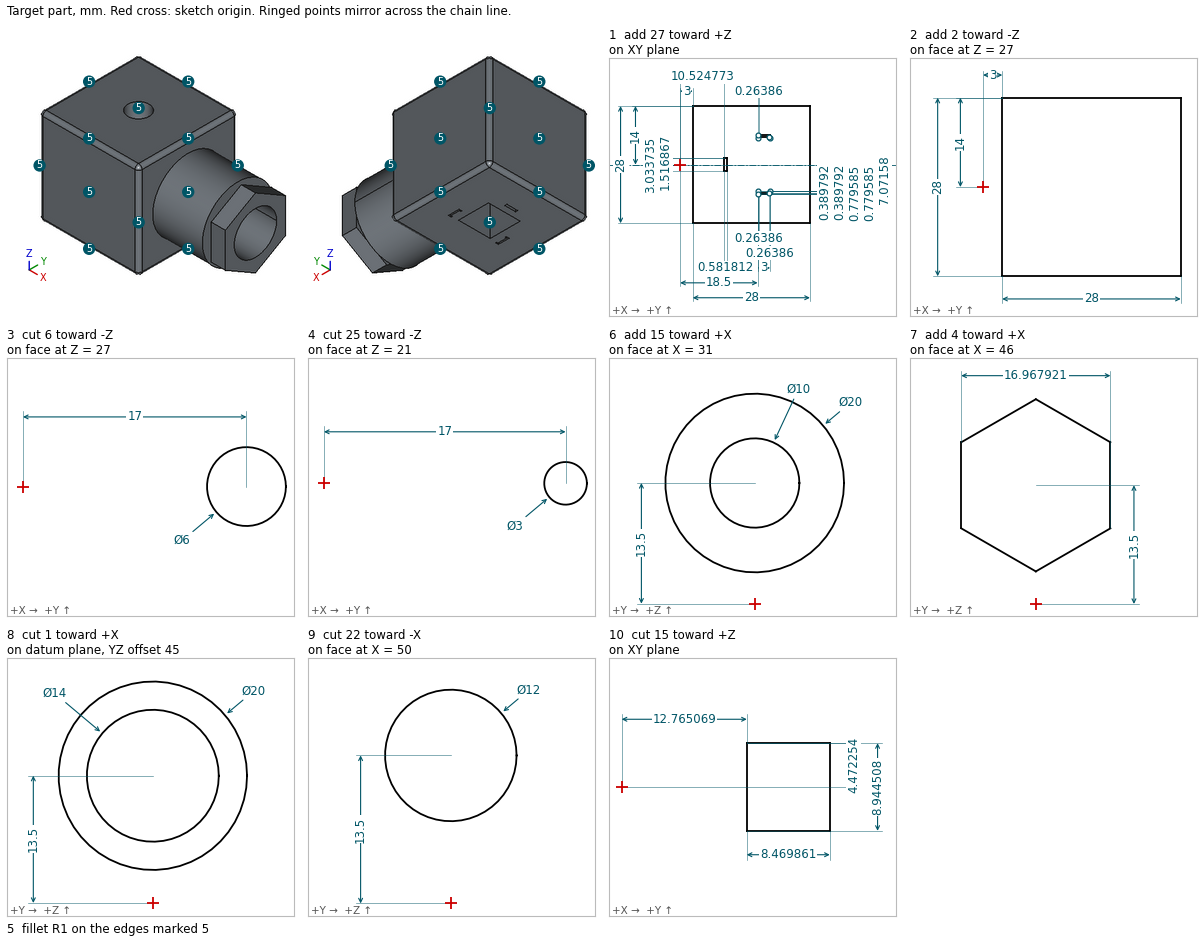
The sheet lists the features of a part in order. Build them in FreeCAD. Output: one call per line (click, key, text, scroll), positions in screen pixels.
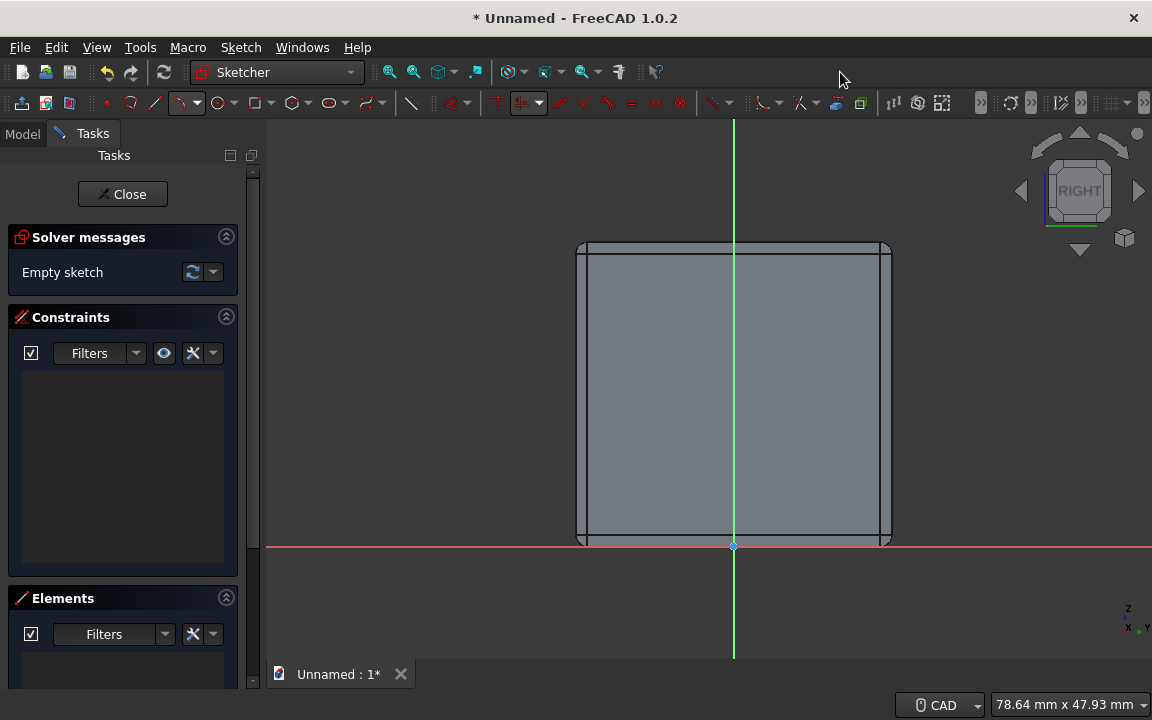
click(218, 104)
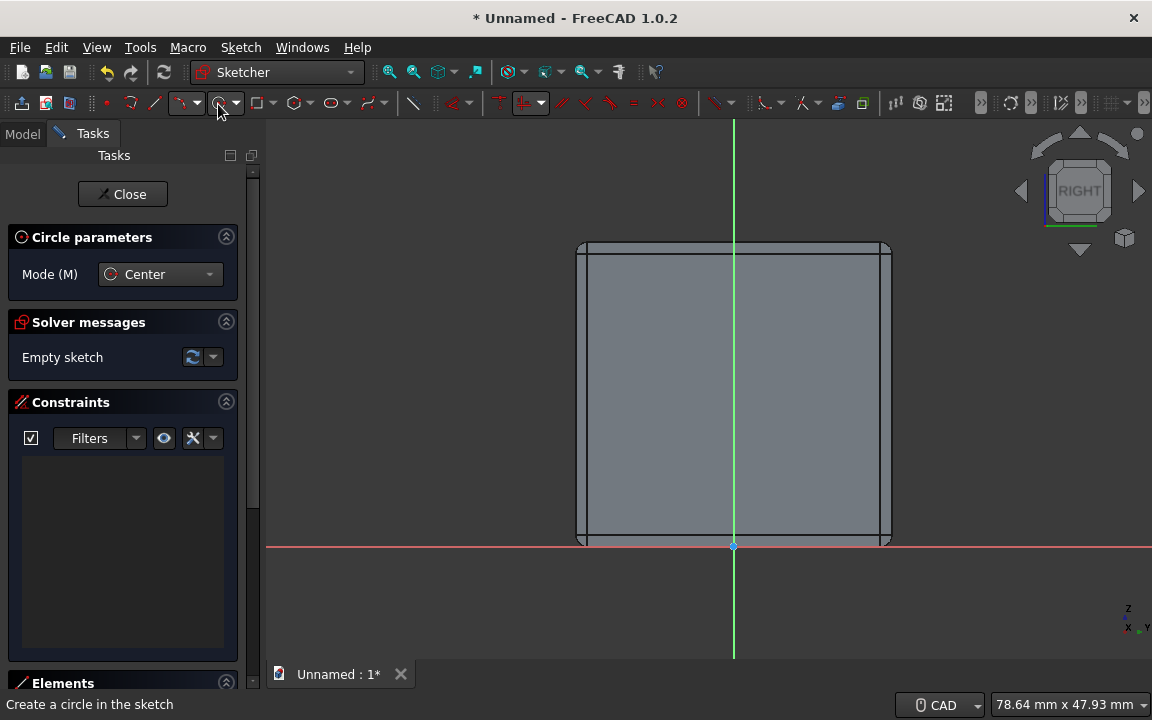
click(734, 394)
click(814, 315)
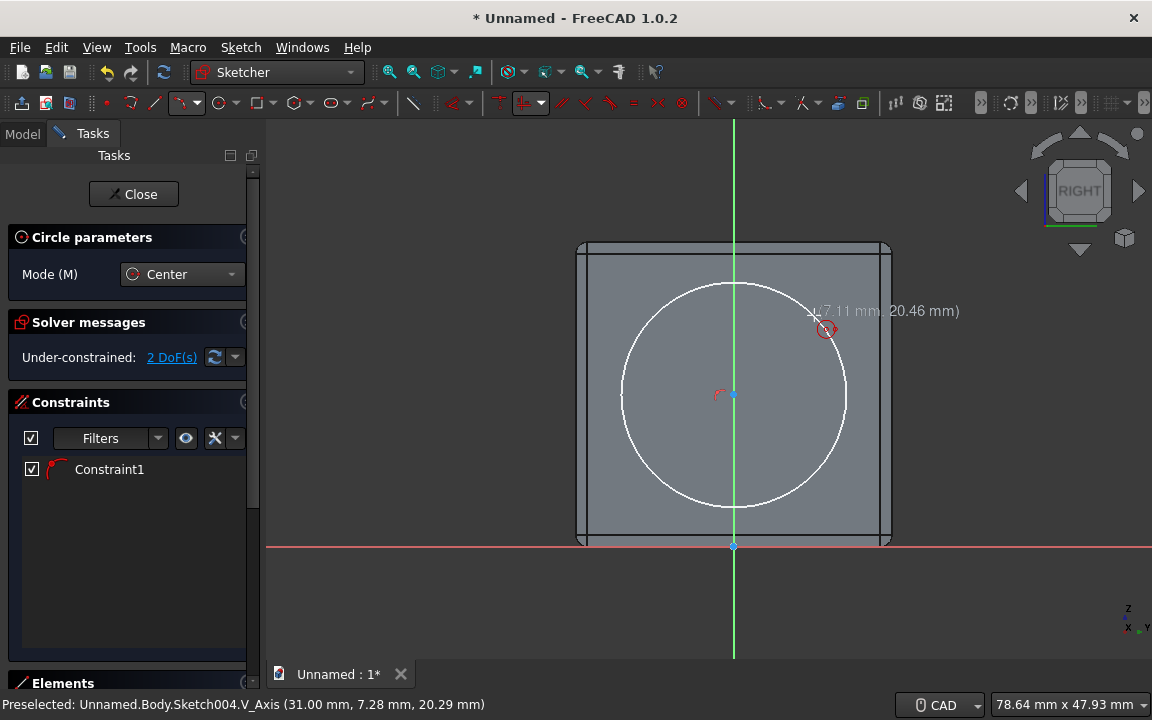
click(734, 395)
click(774, 355)
key(Escape)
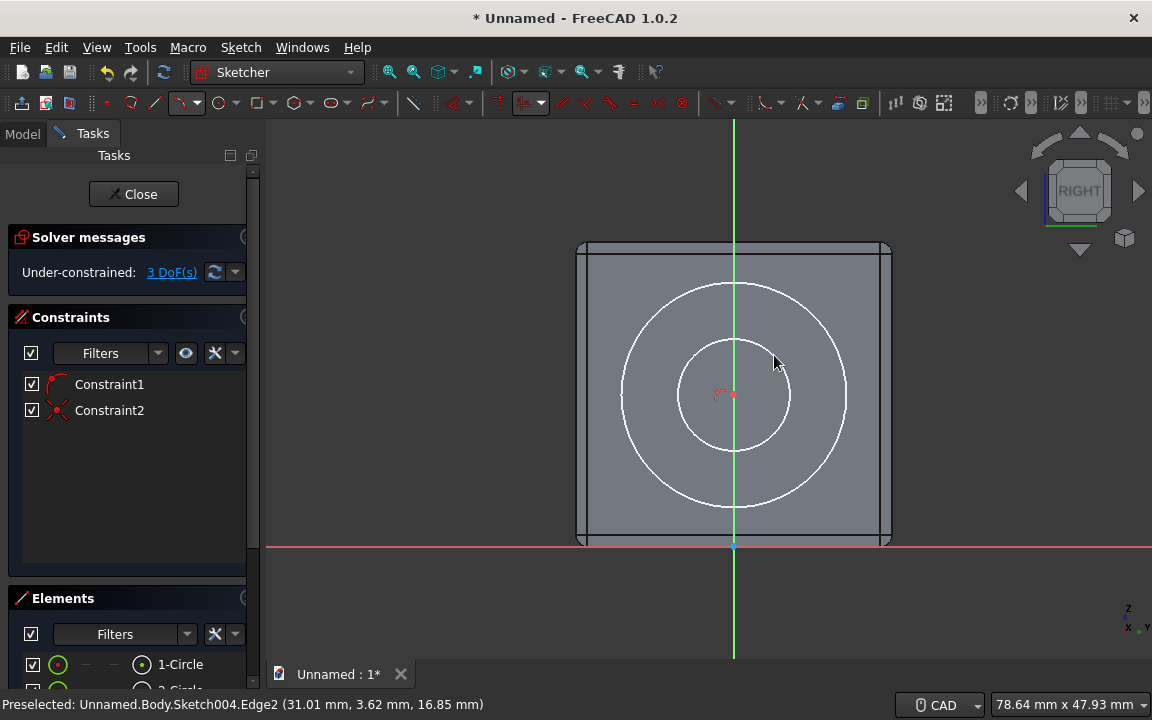
click(452, 104)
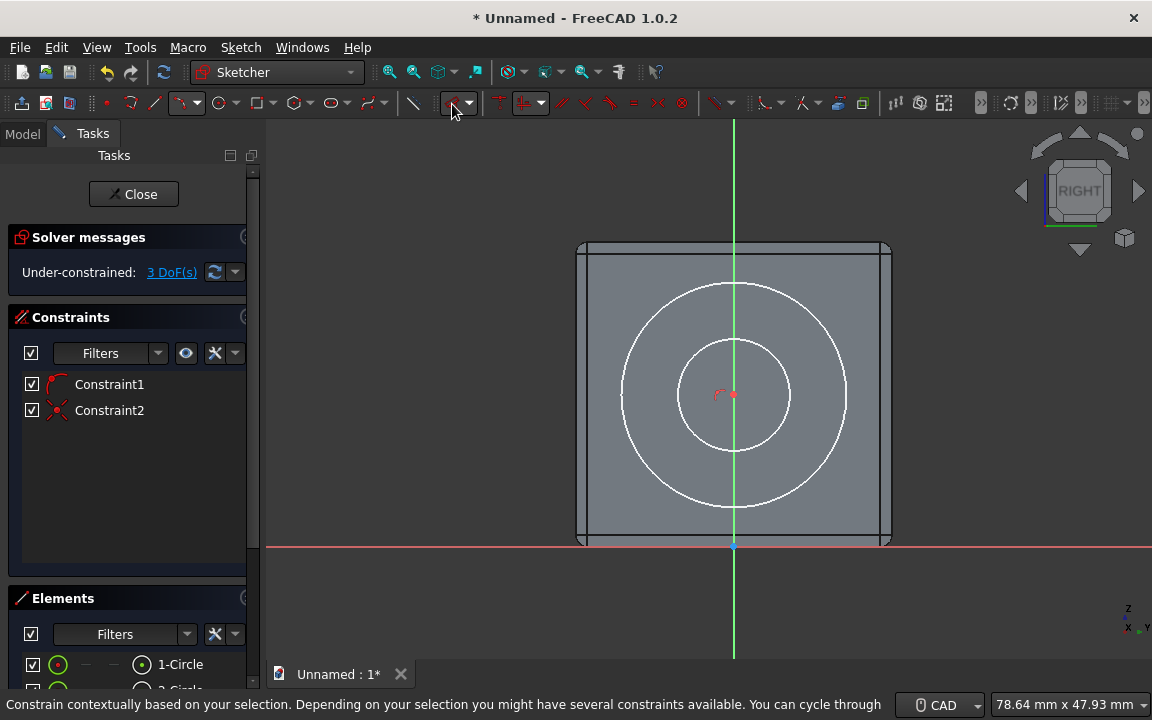
click(813, 315)
click(835, 292)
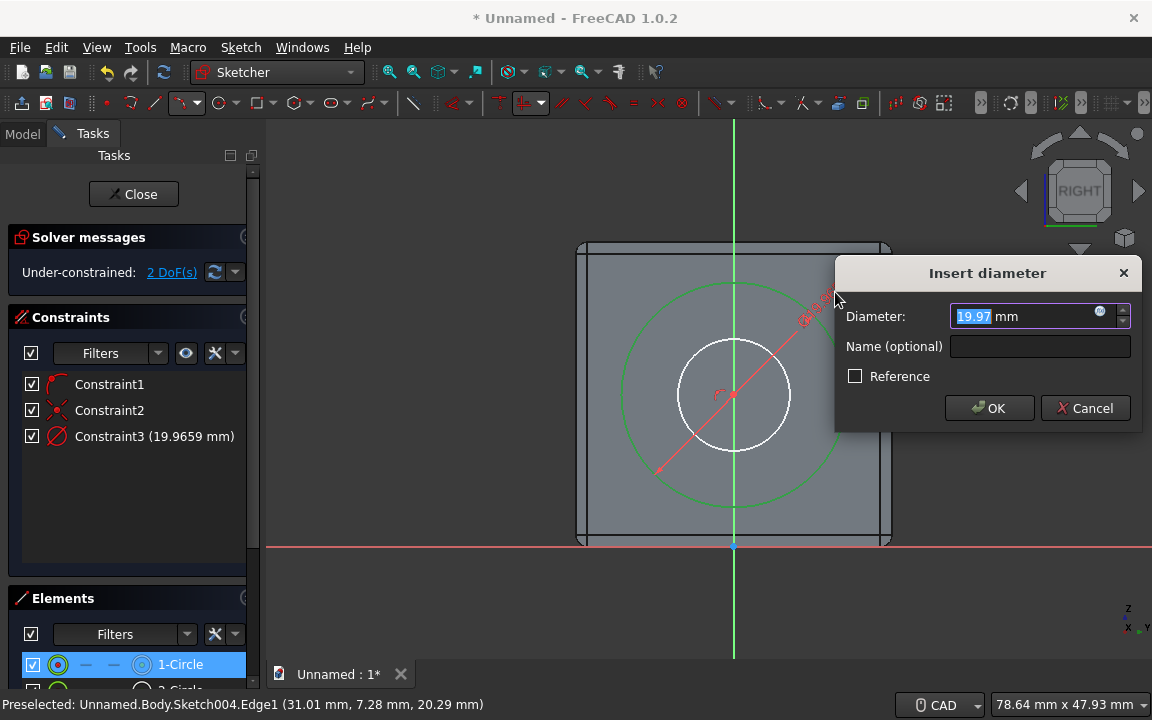
text(20)
key(Return)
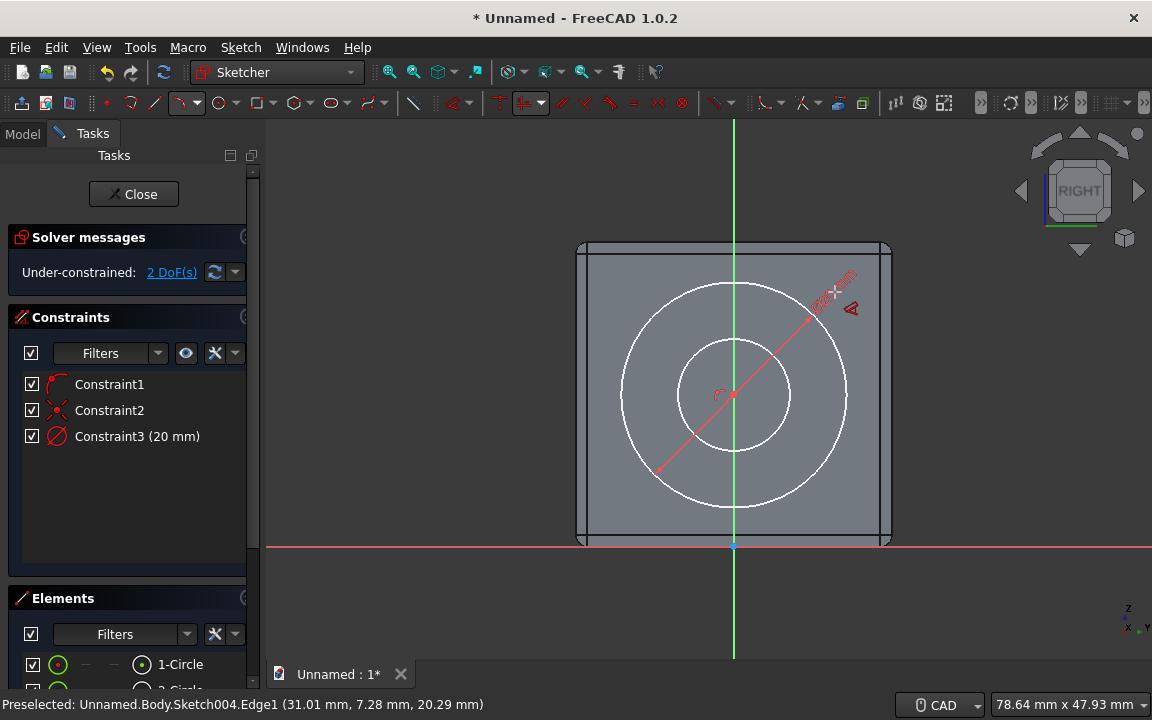
click(773, 355)
click(795, 332)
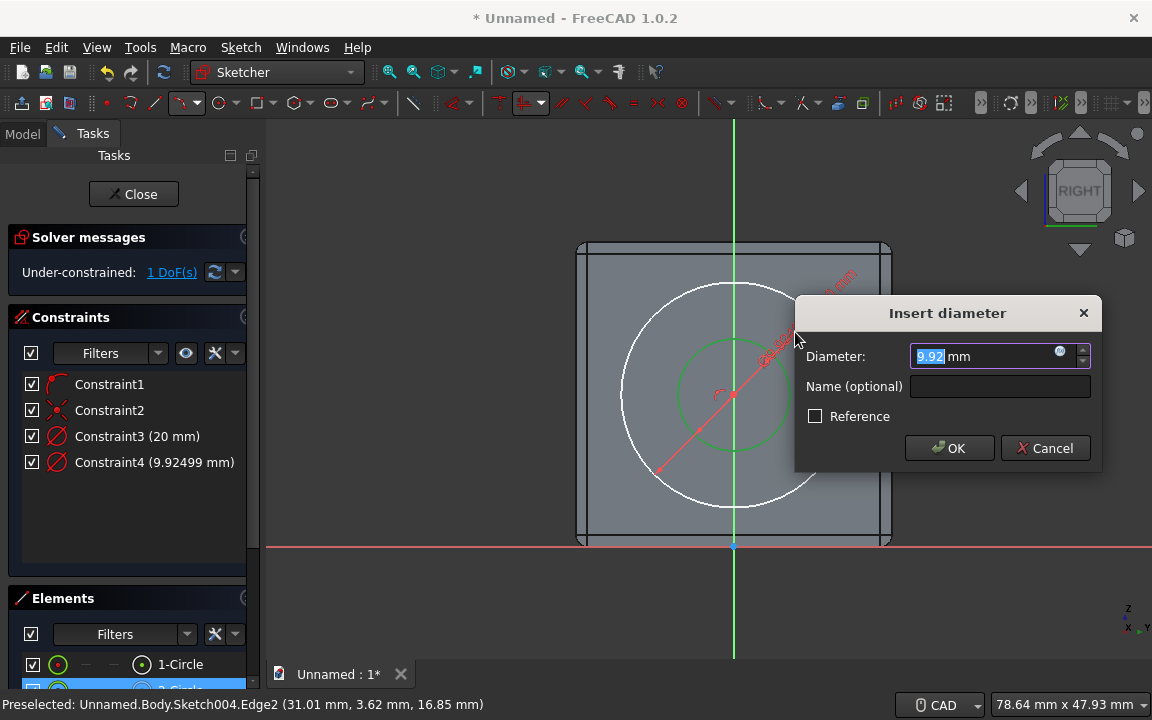
text(10)
key(Return)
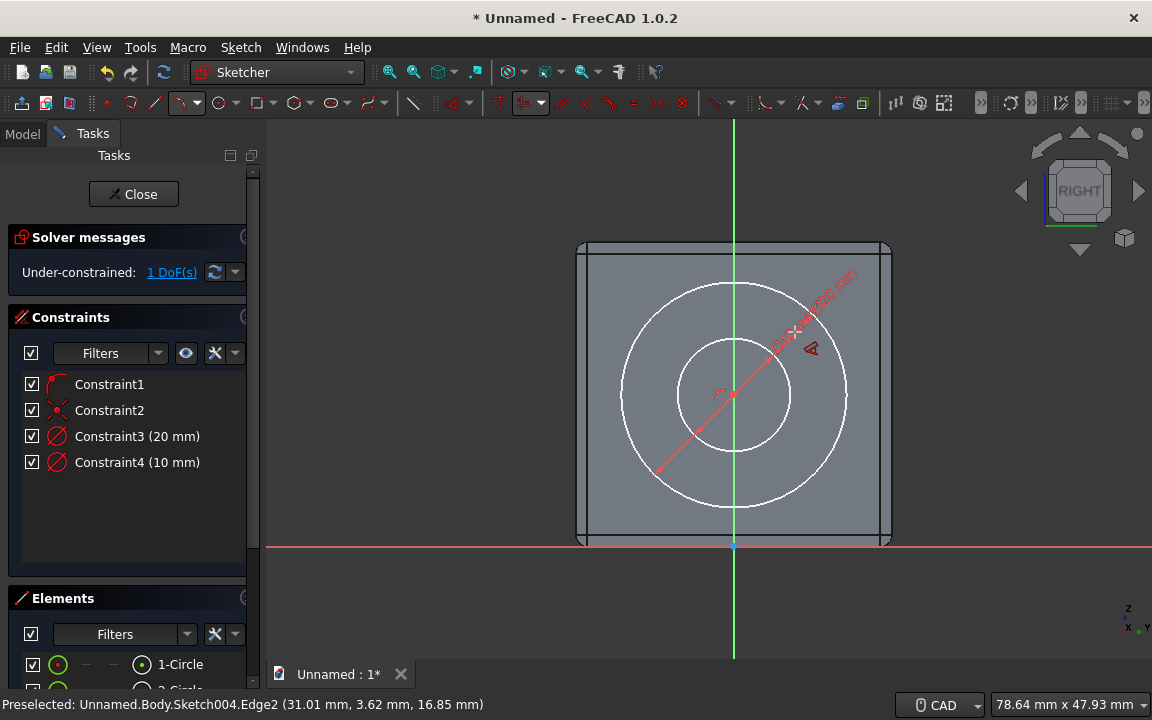
click(734, 395)
click(768, 471)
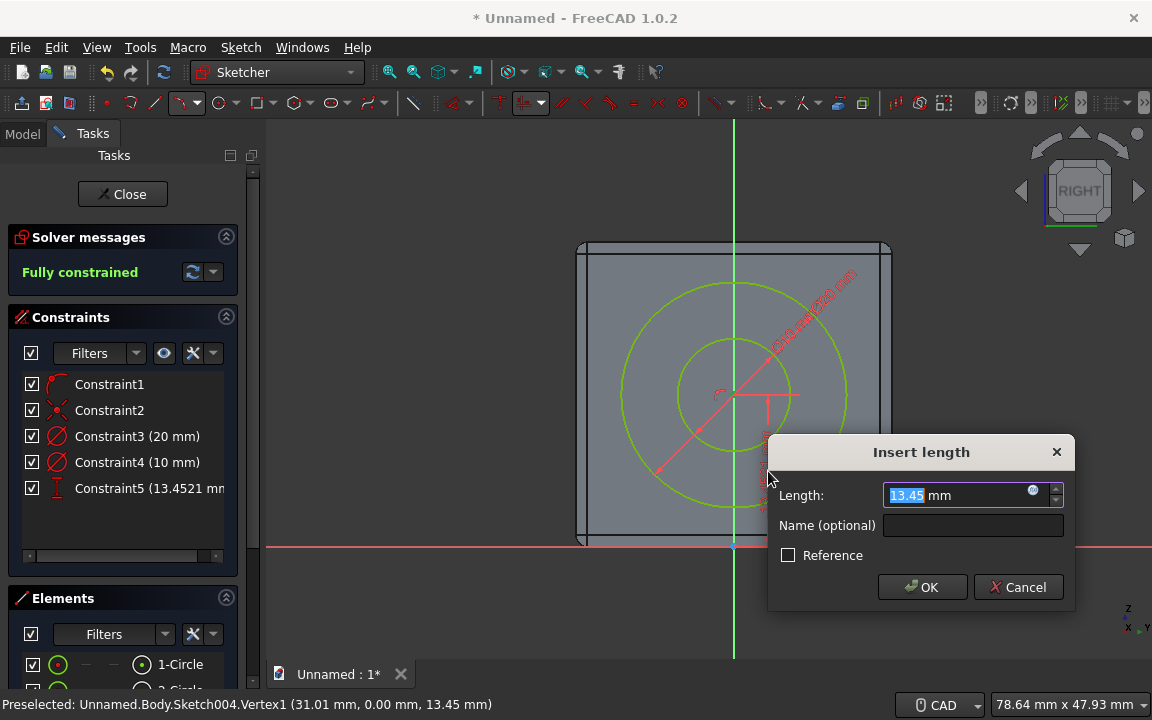
text(13.5)
key(Return)
key(Escape)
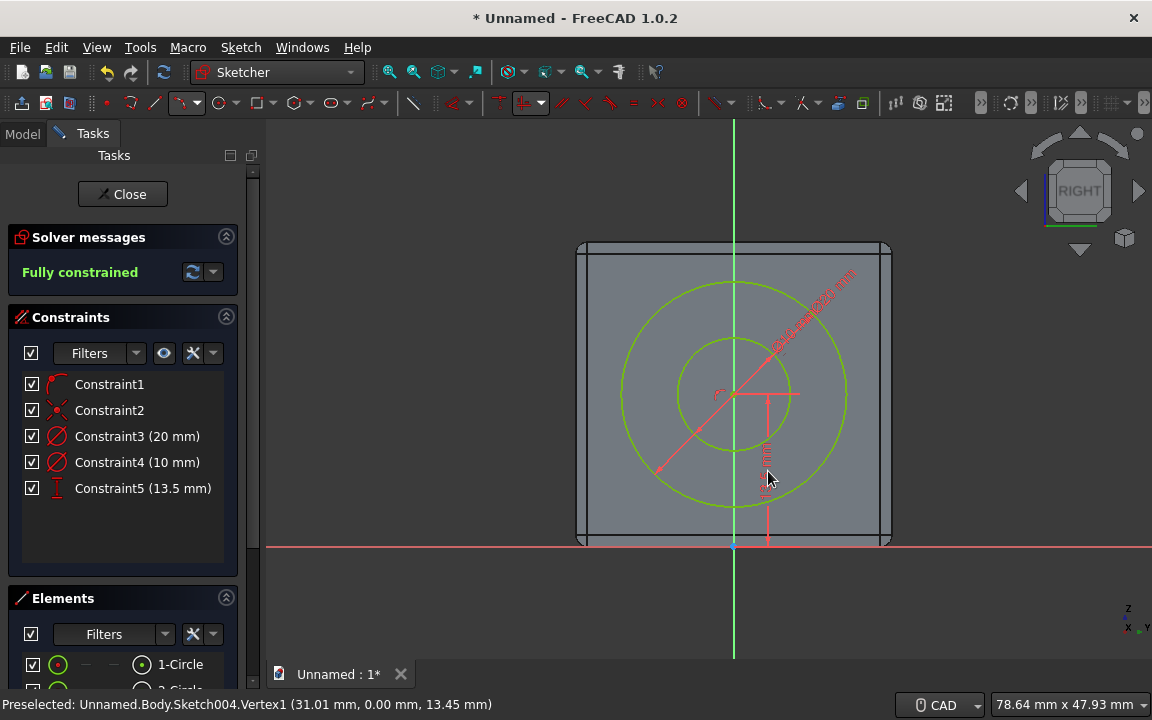
click(123, 194)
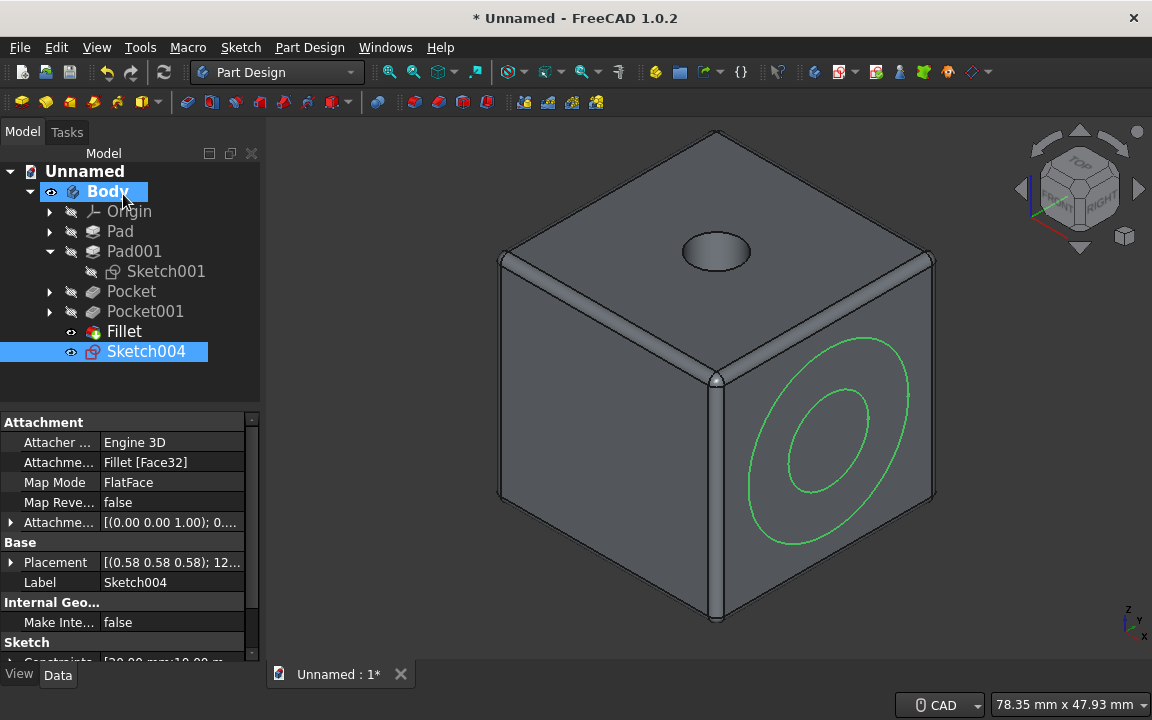
click(22, 102)